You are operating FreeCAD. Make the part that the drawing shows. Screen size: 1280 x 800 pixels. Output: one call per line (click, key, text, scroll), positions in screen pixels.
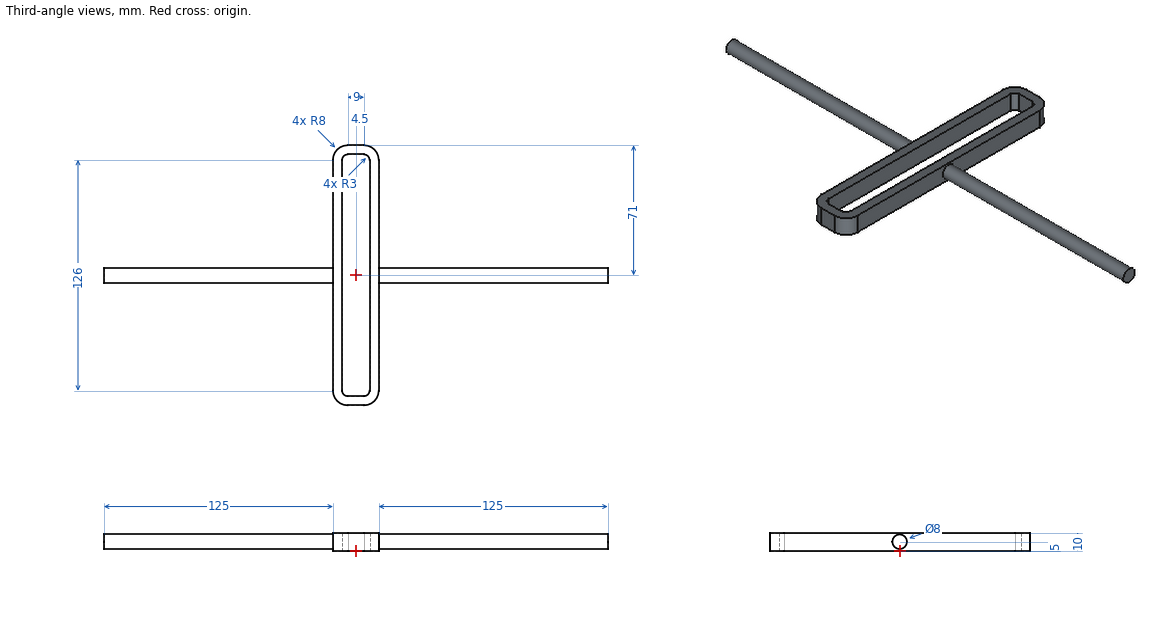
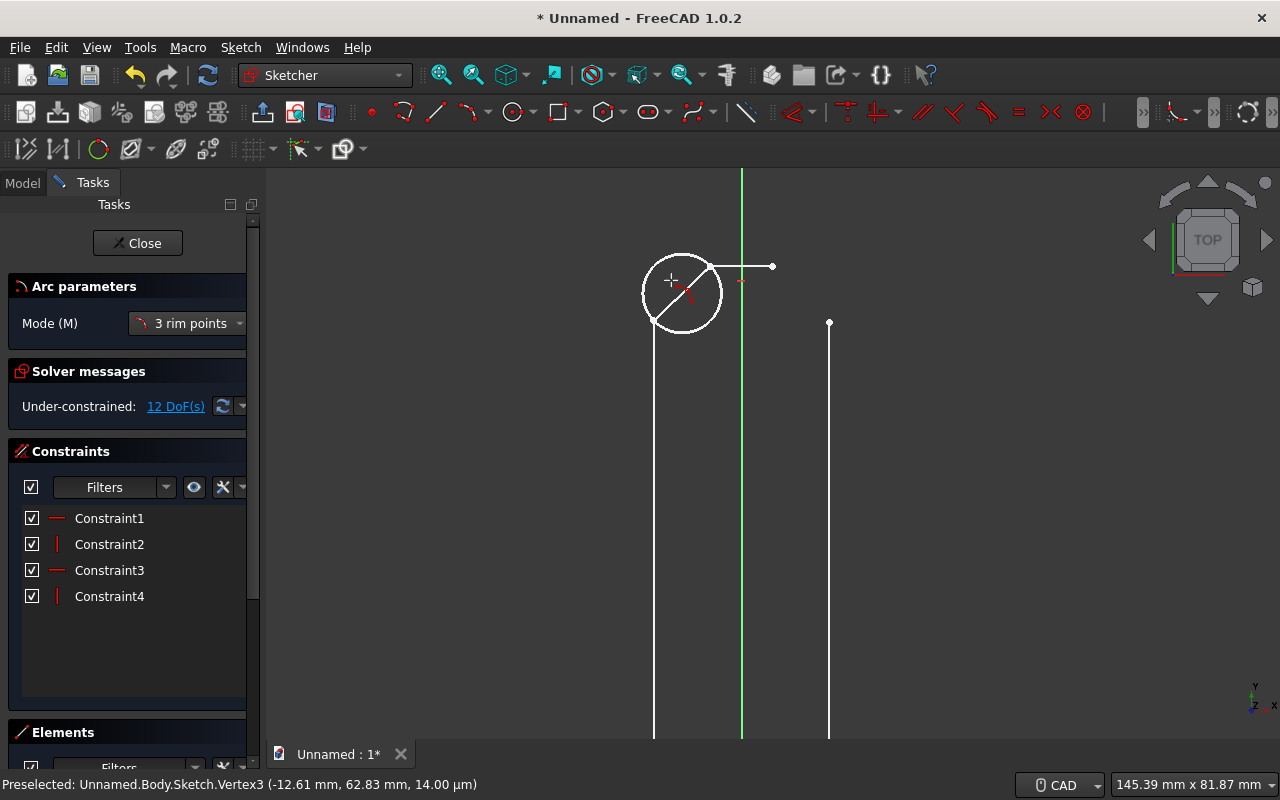
click(671, 280)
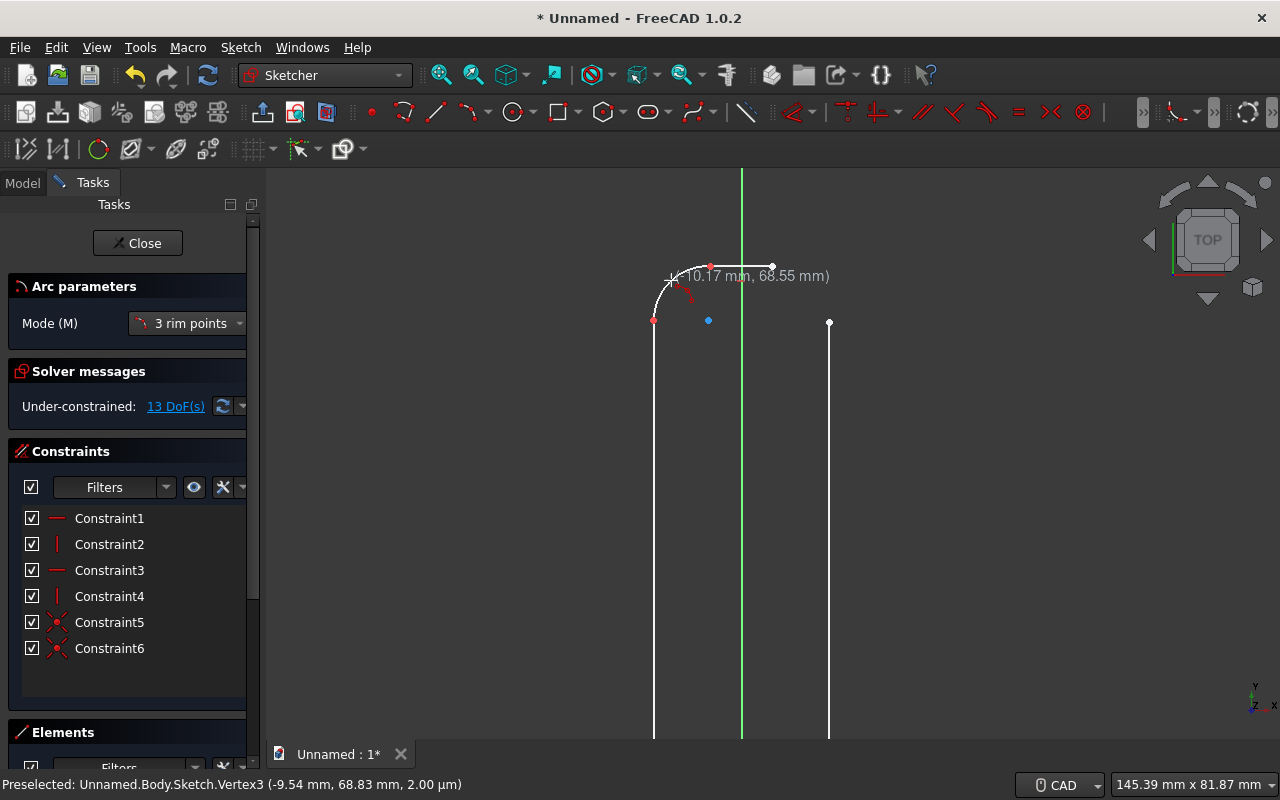
scroll(683, 276, down, 5)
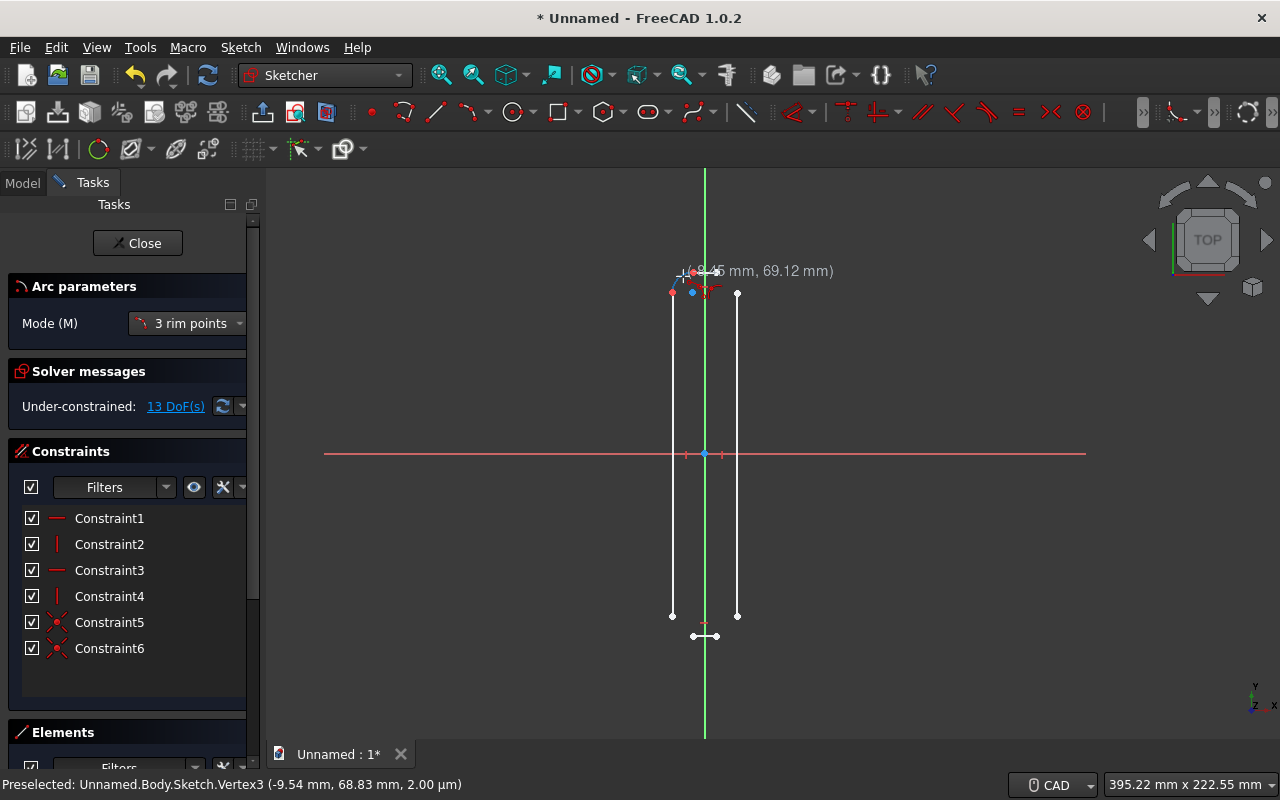
click(673, 616)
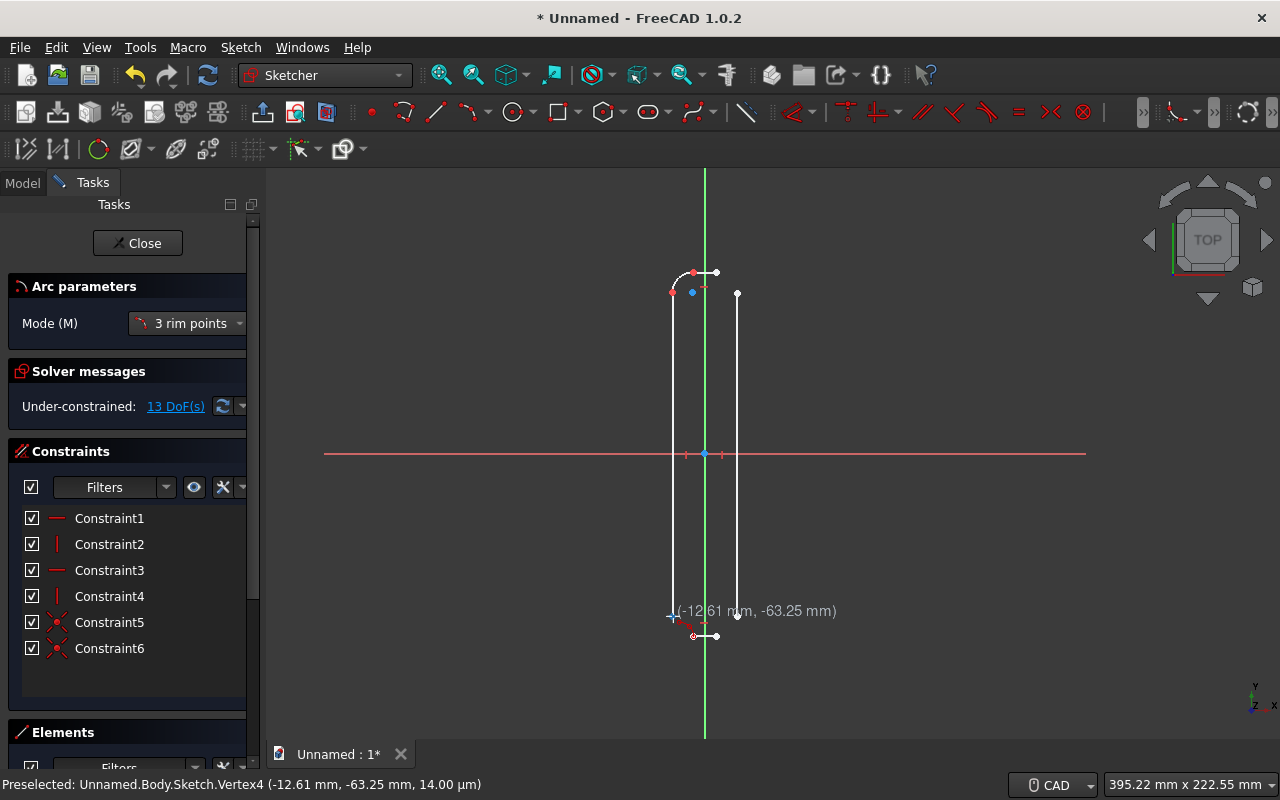
scroll(693, 636, up, 2)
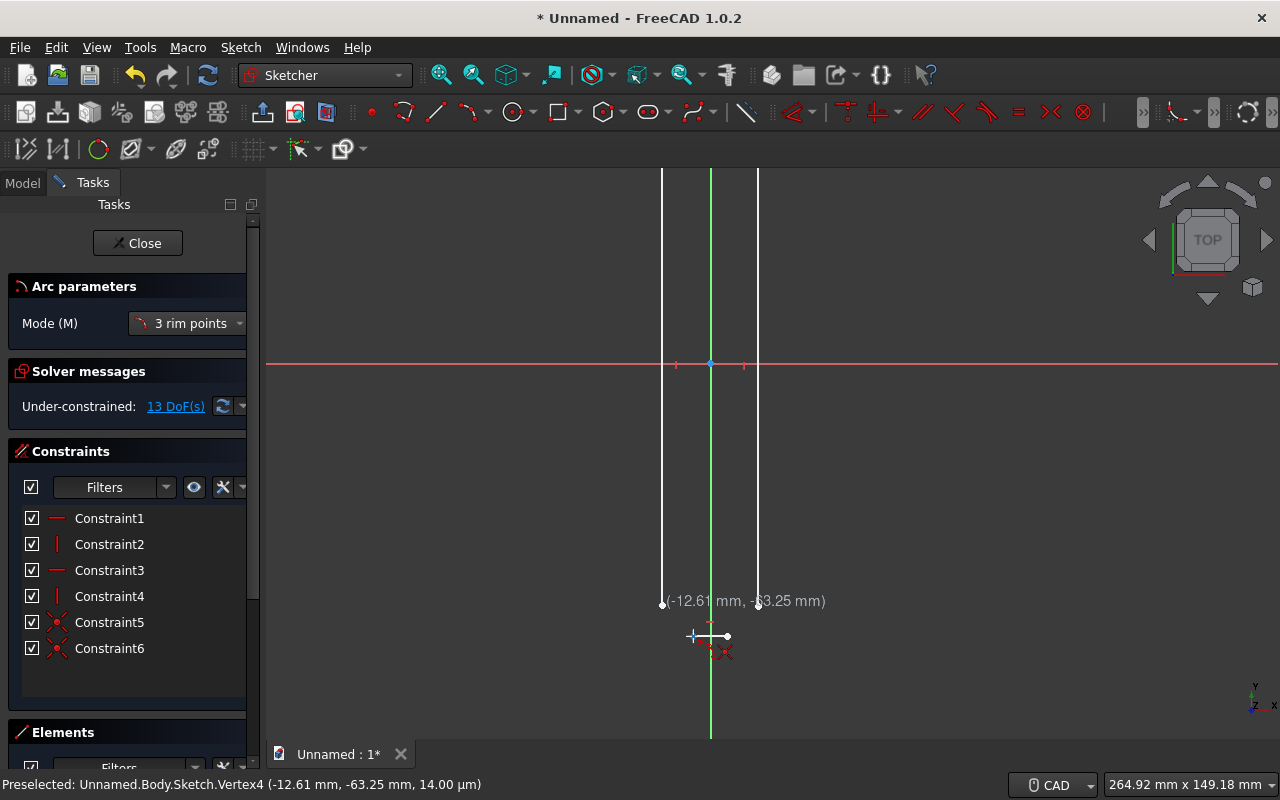
click(693, 636)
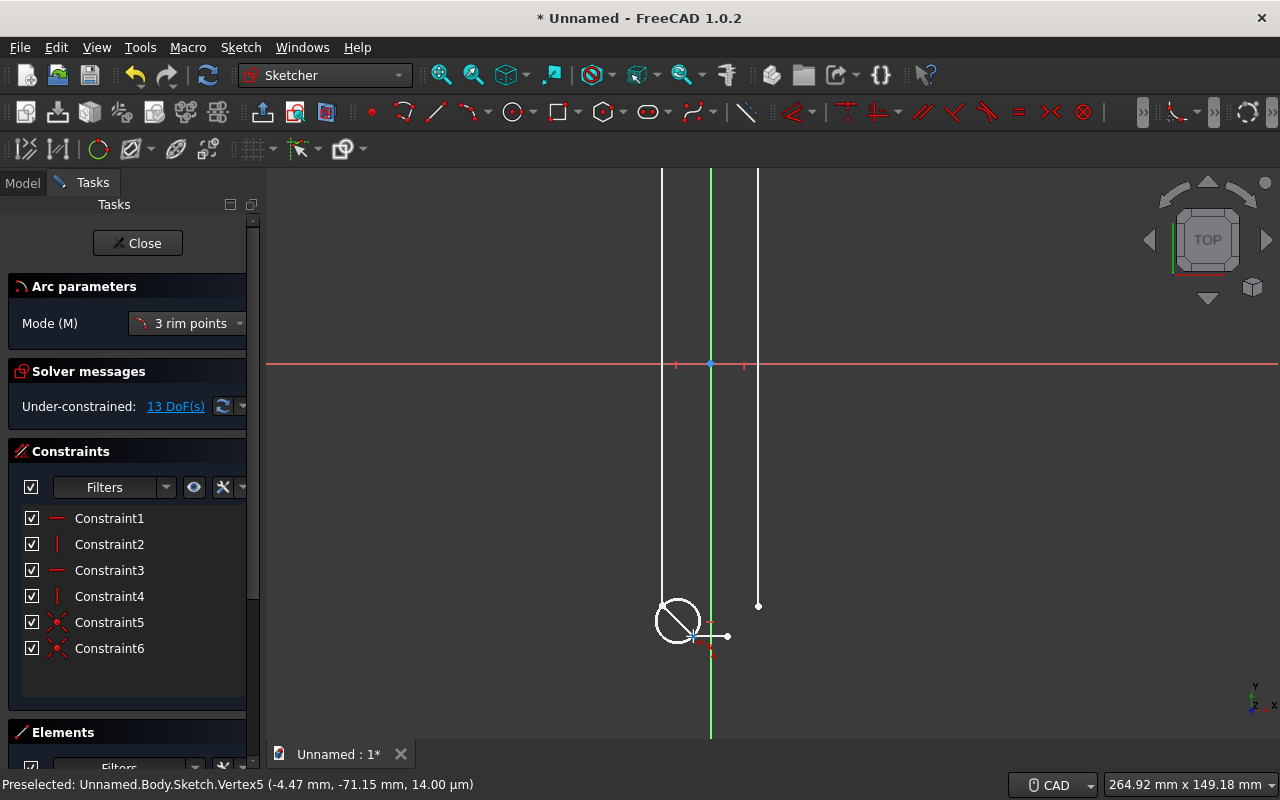
scroll(672, 627, up, 3)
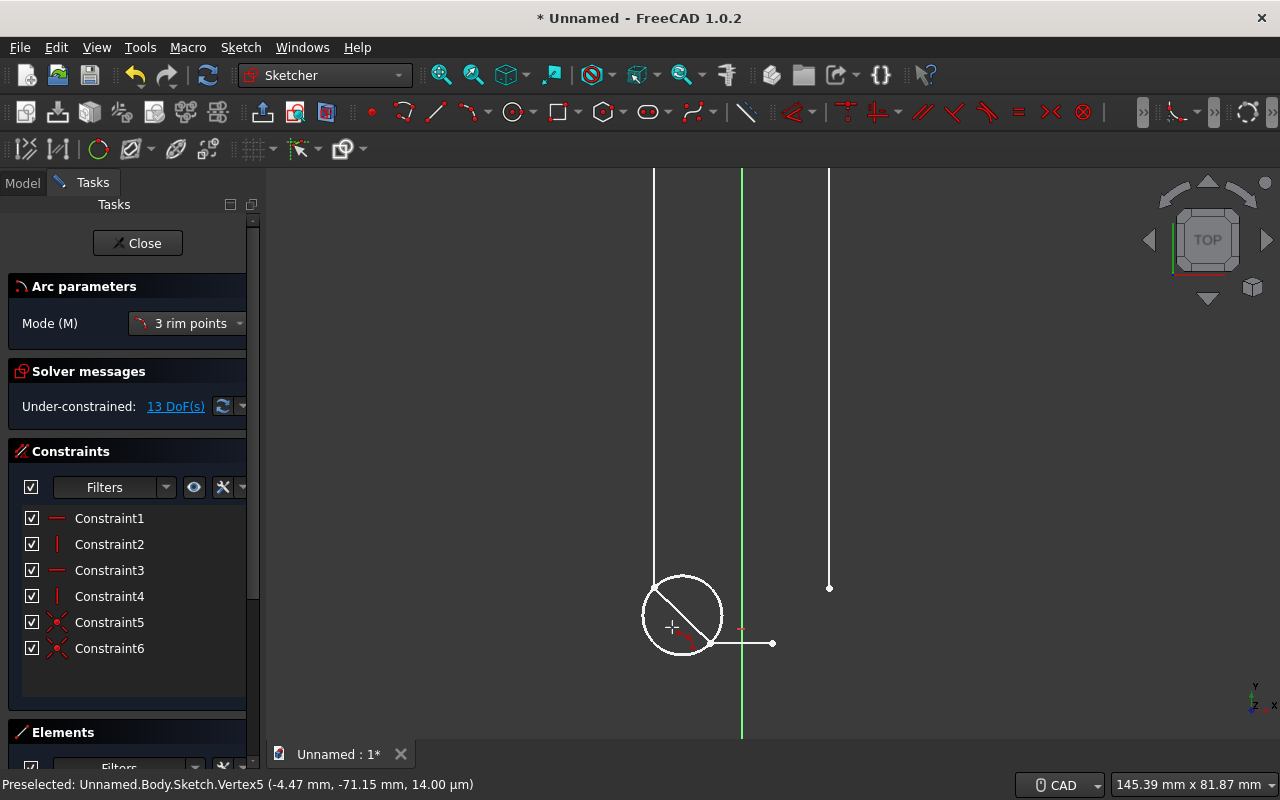
click(671, 626)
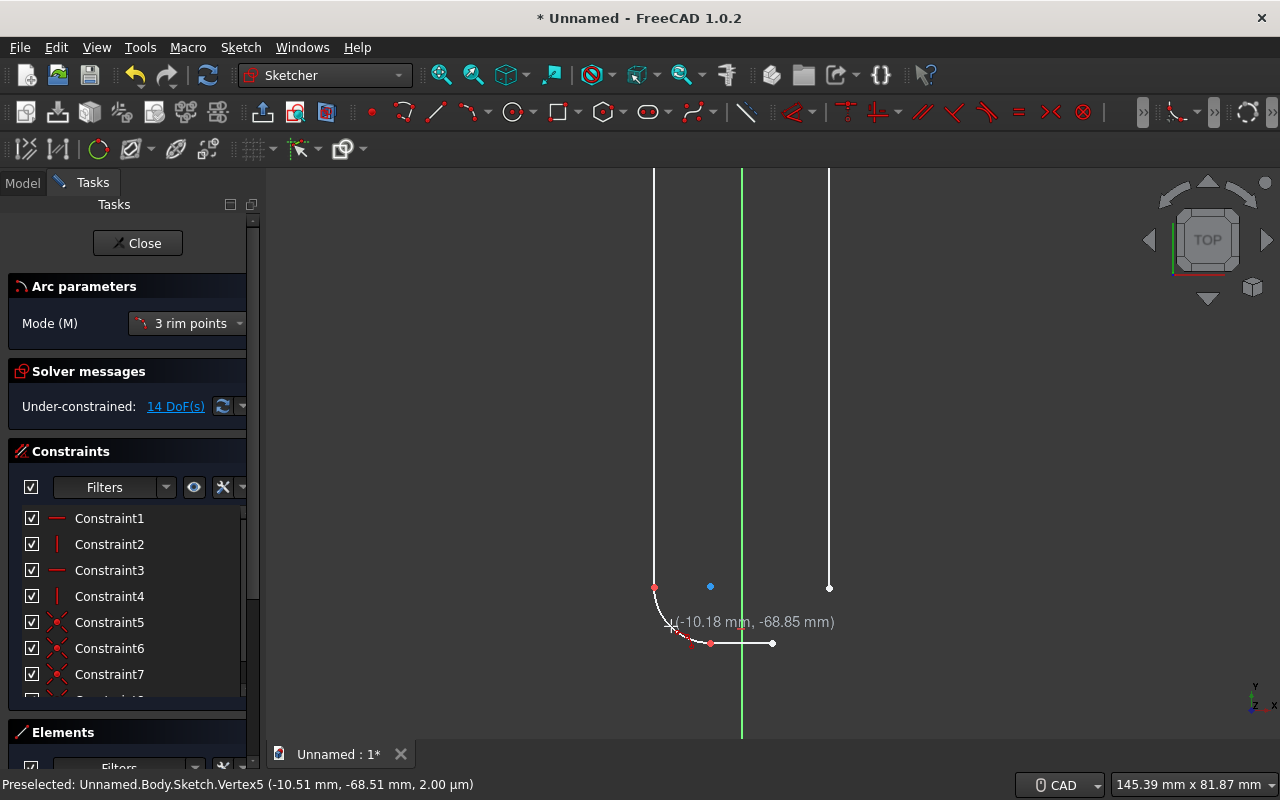
click(773, 643)
click(829, 588)
click(813, 626)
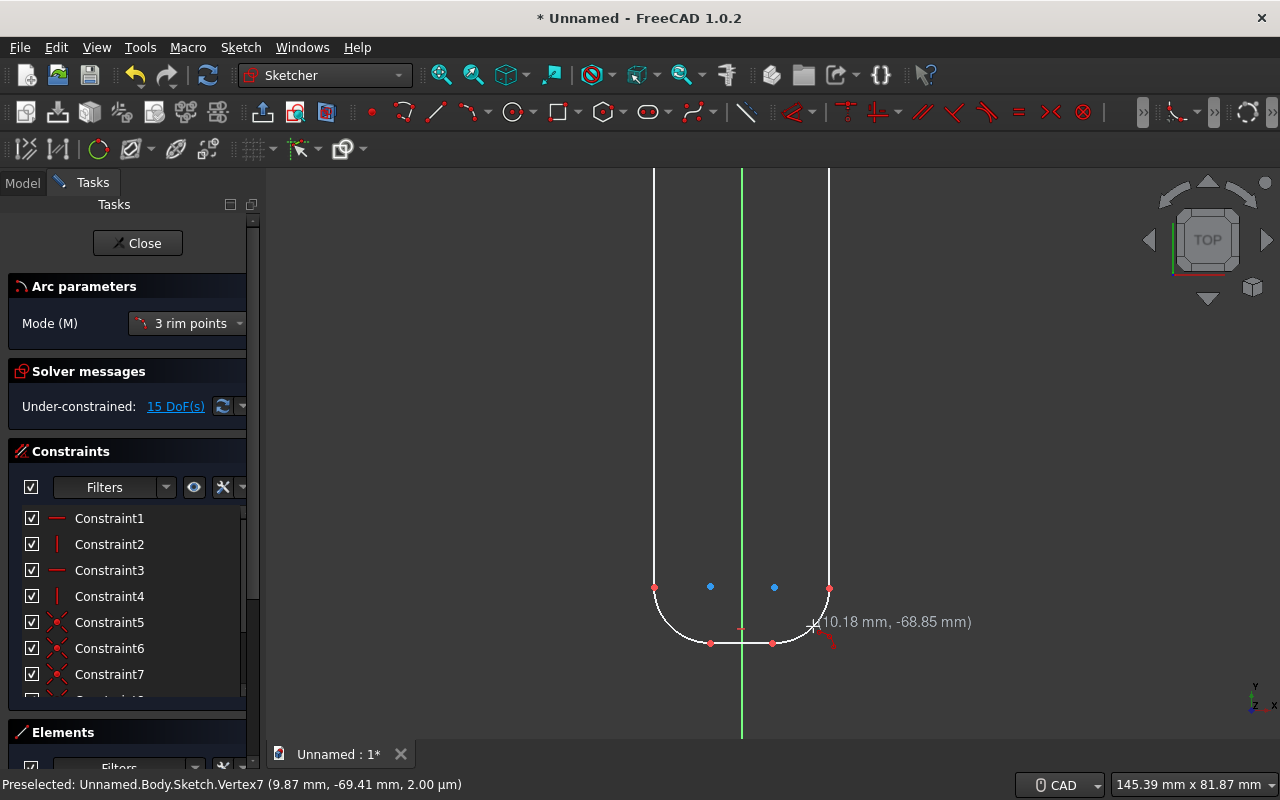
scroll(683, 632, down, 5)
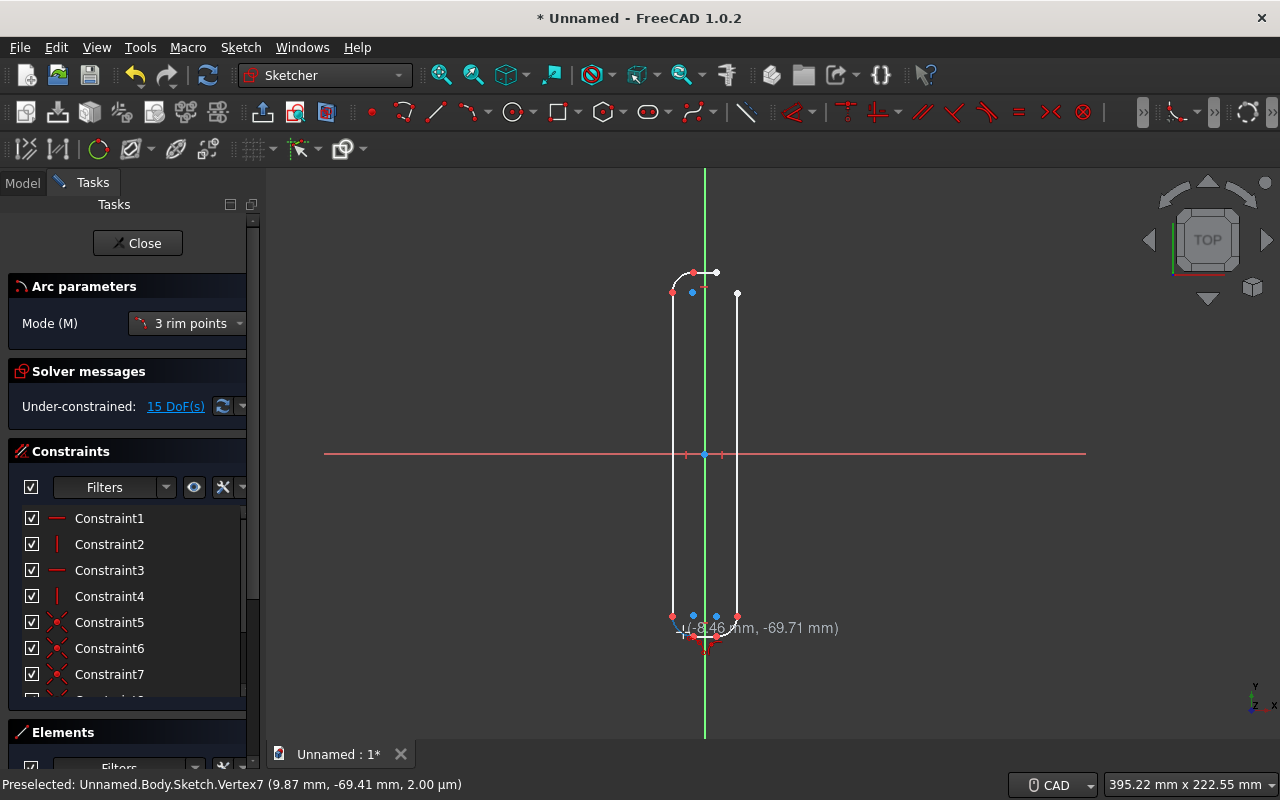
click(737, 293)